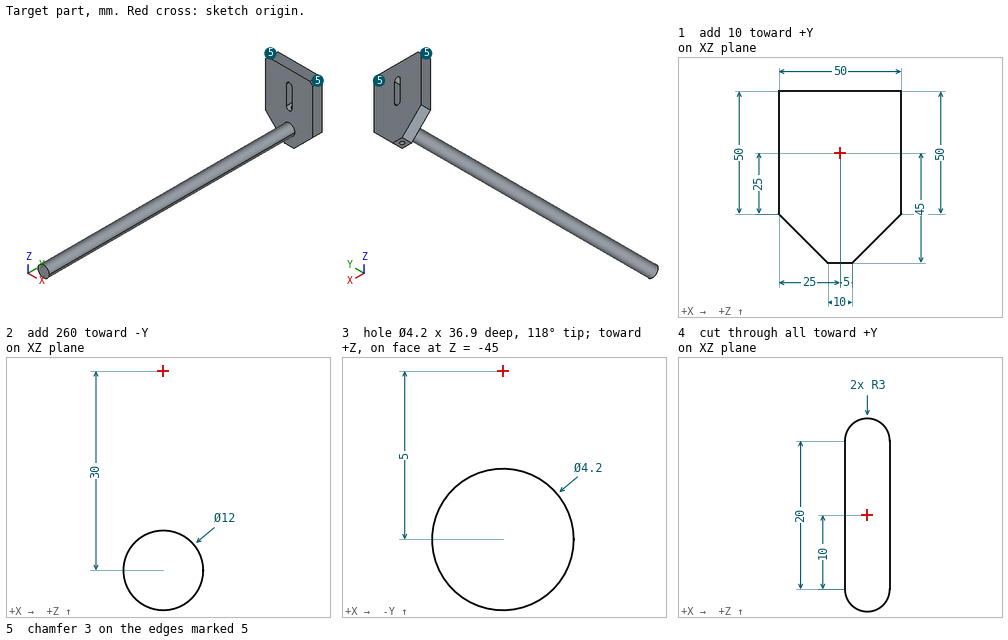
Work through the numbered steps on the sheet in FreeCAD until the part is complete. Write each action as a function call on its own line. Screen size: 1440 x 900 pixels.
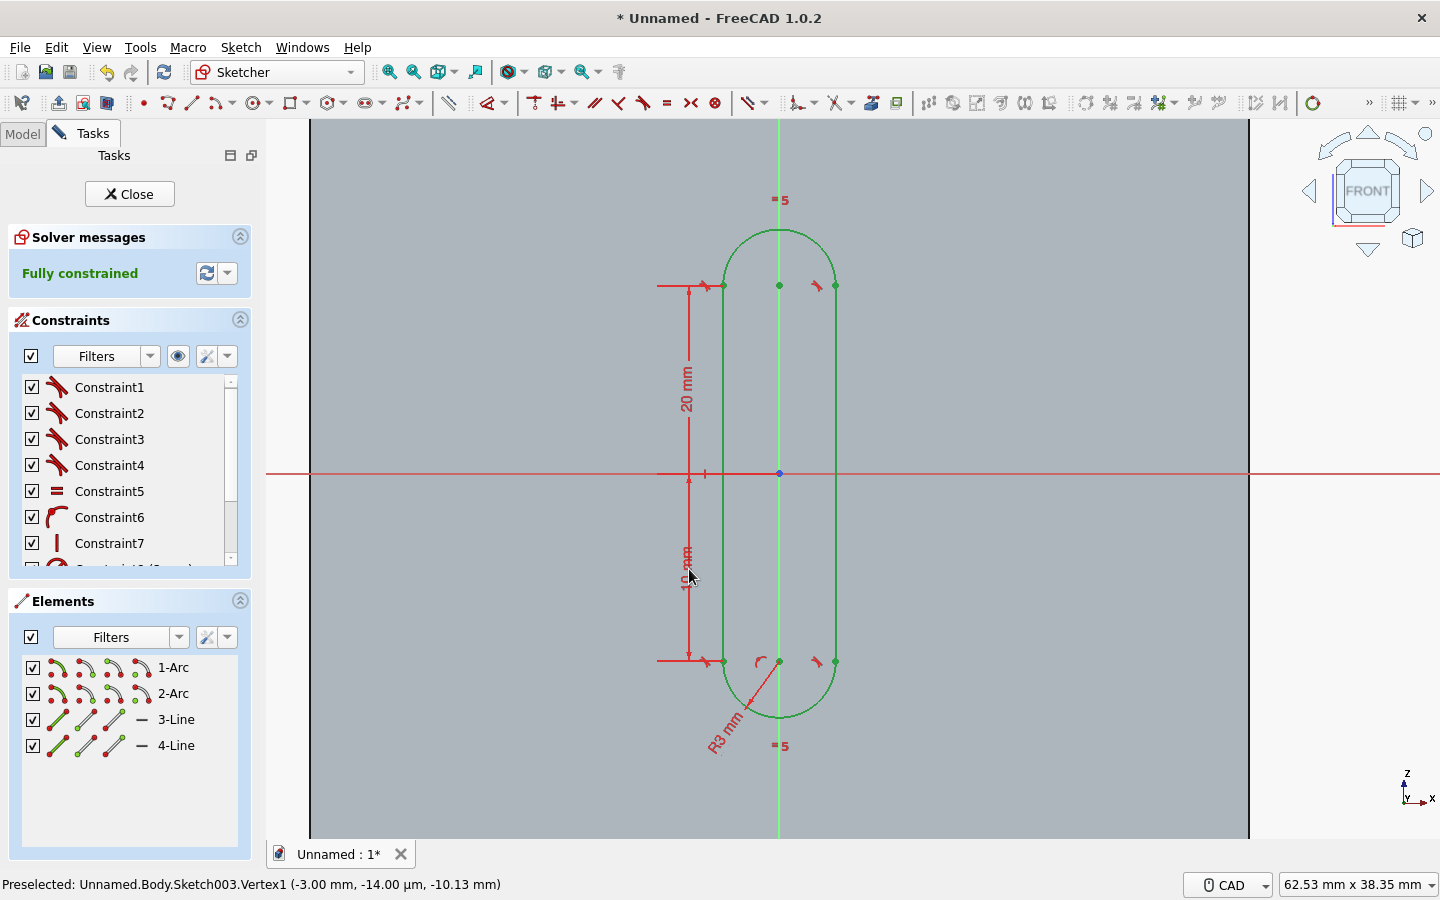
click(130, 194)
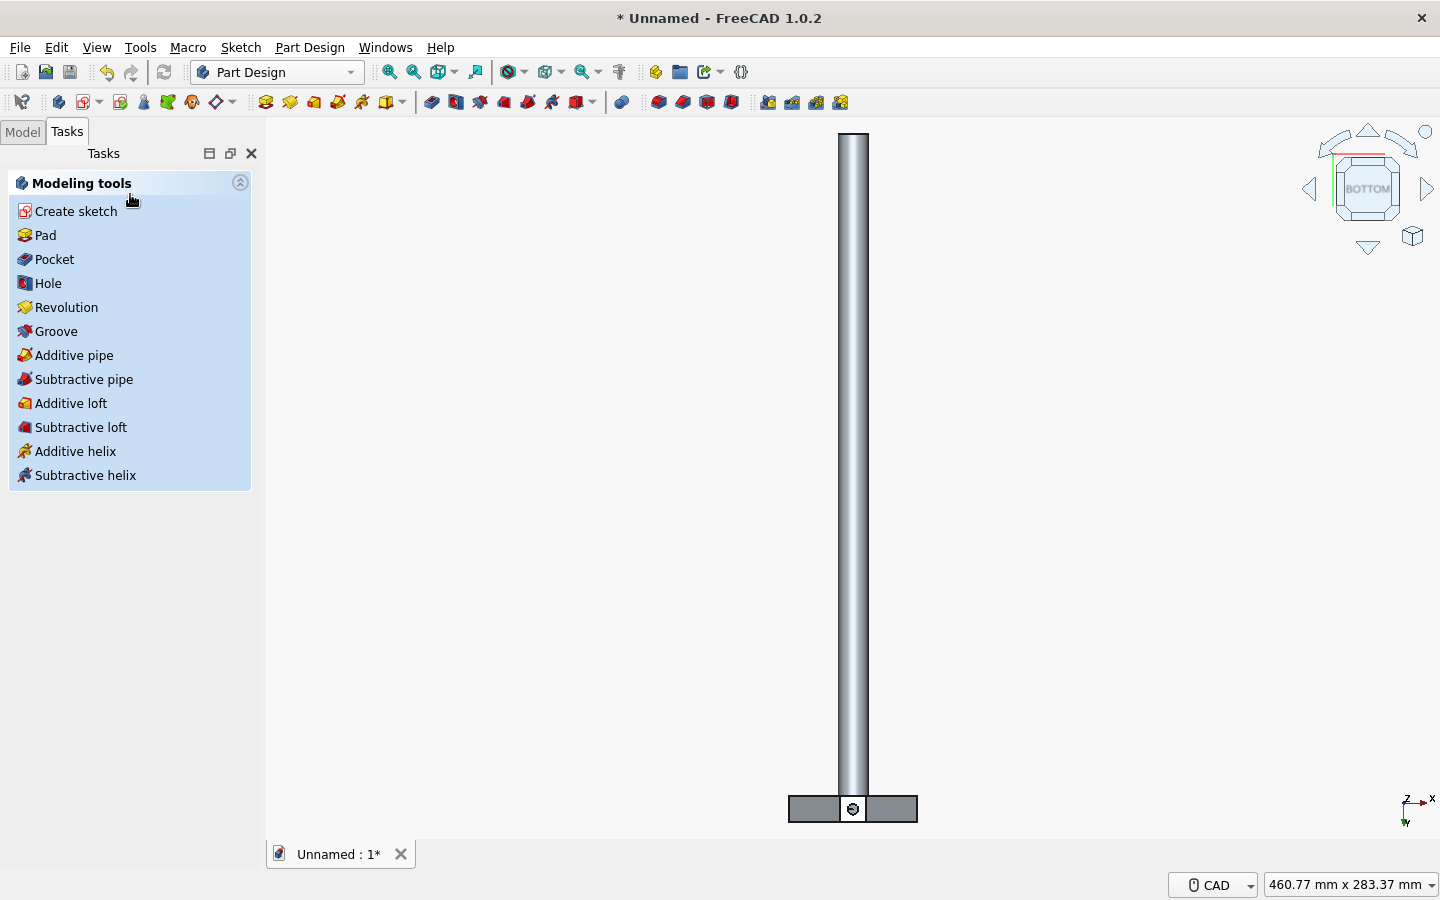
click(432, 102)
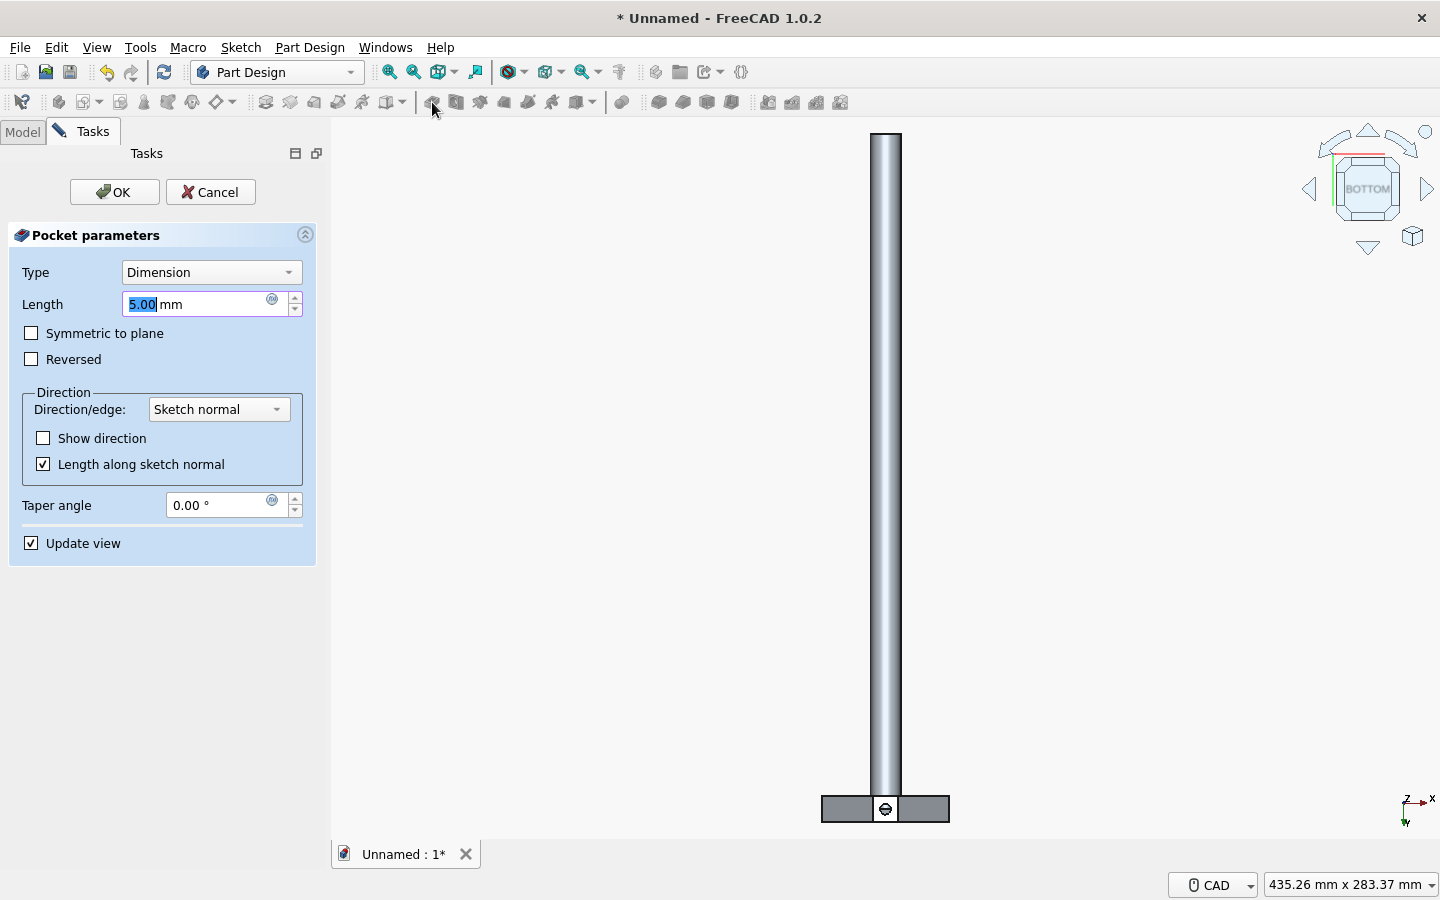
click(212, 272)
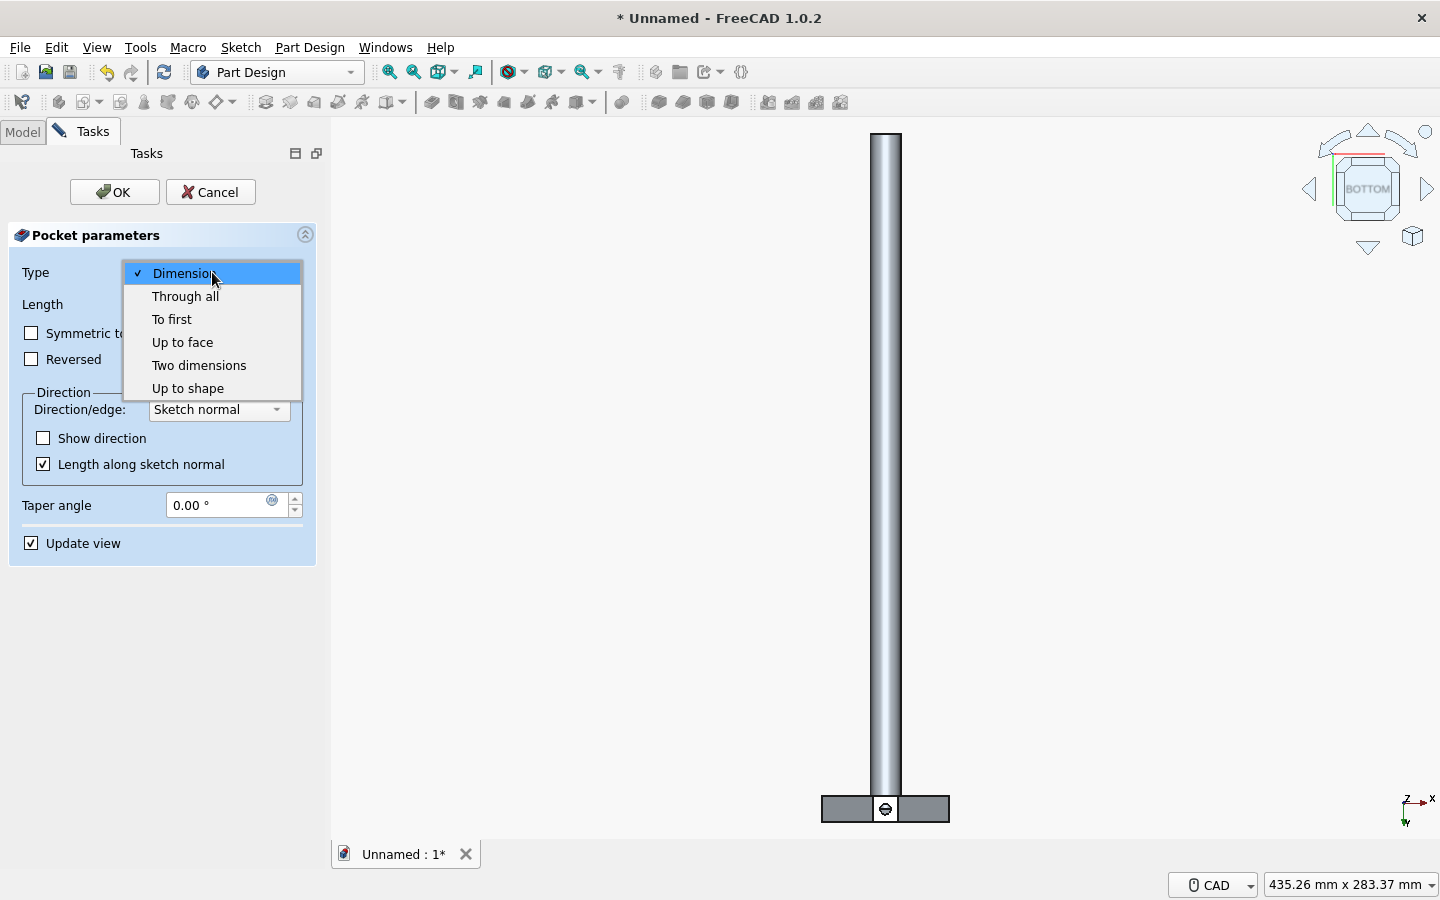
click(212, 296)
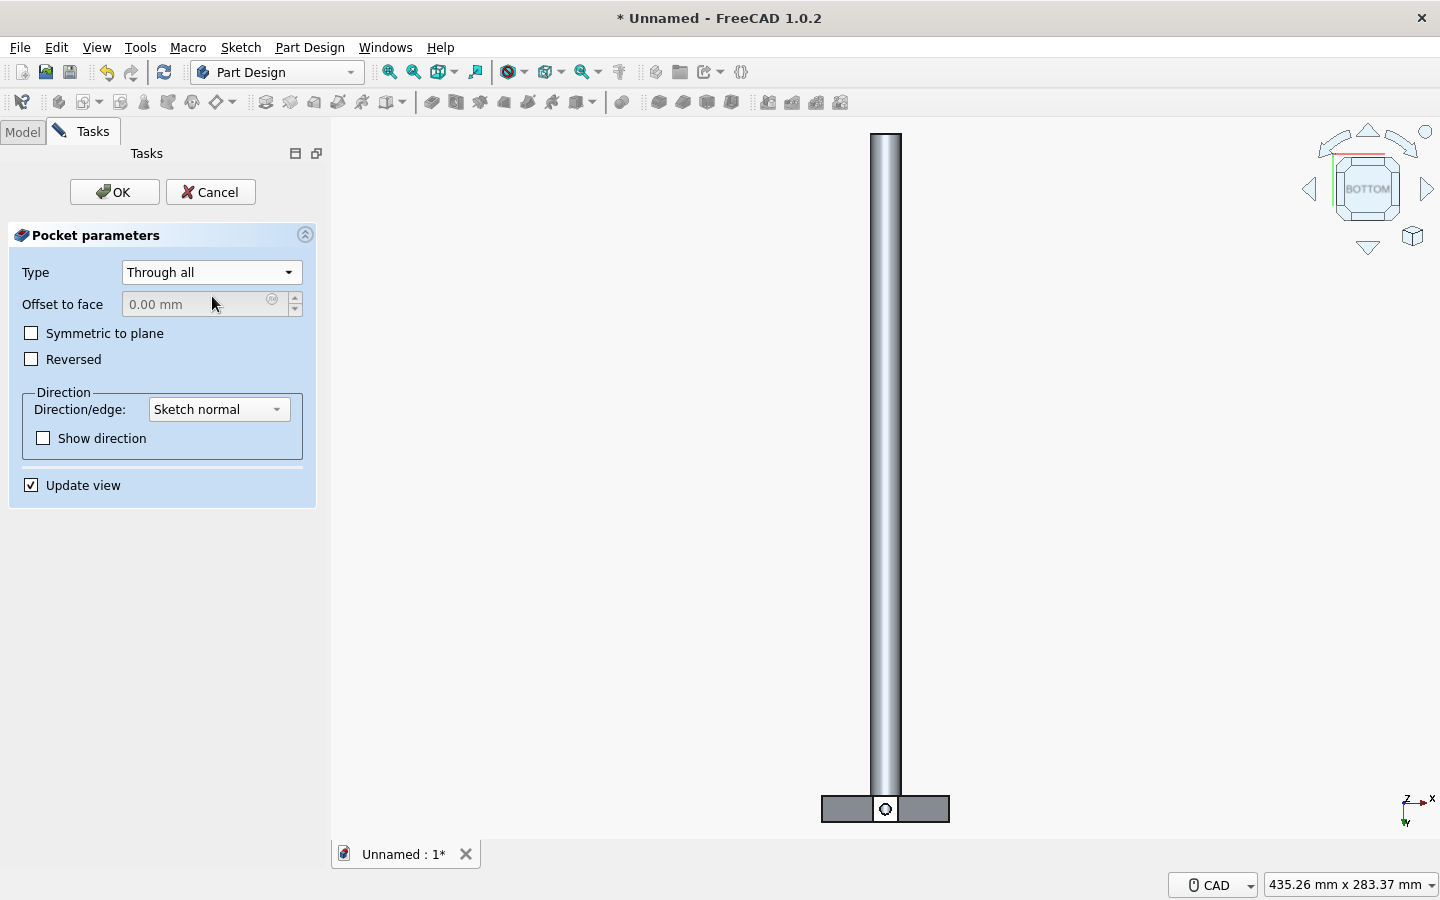
click(115, 192)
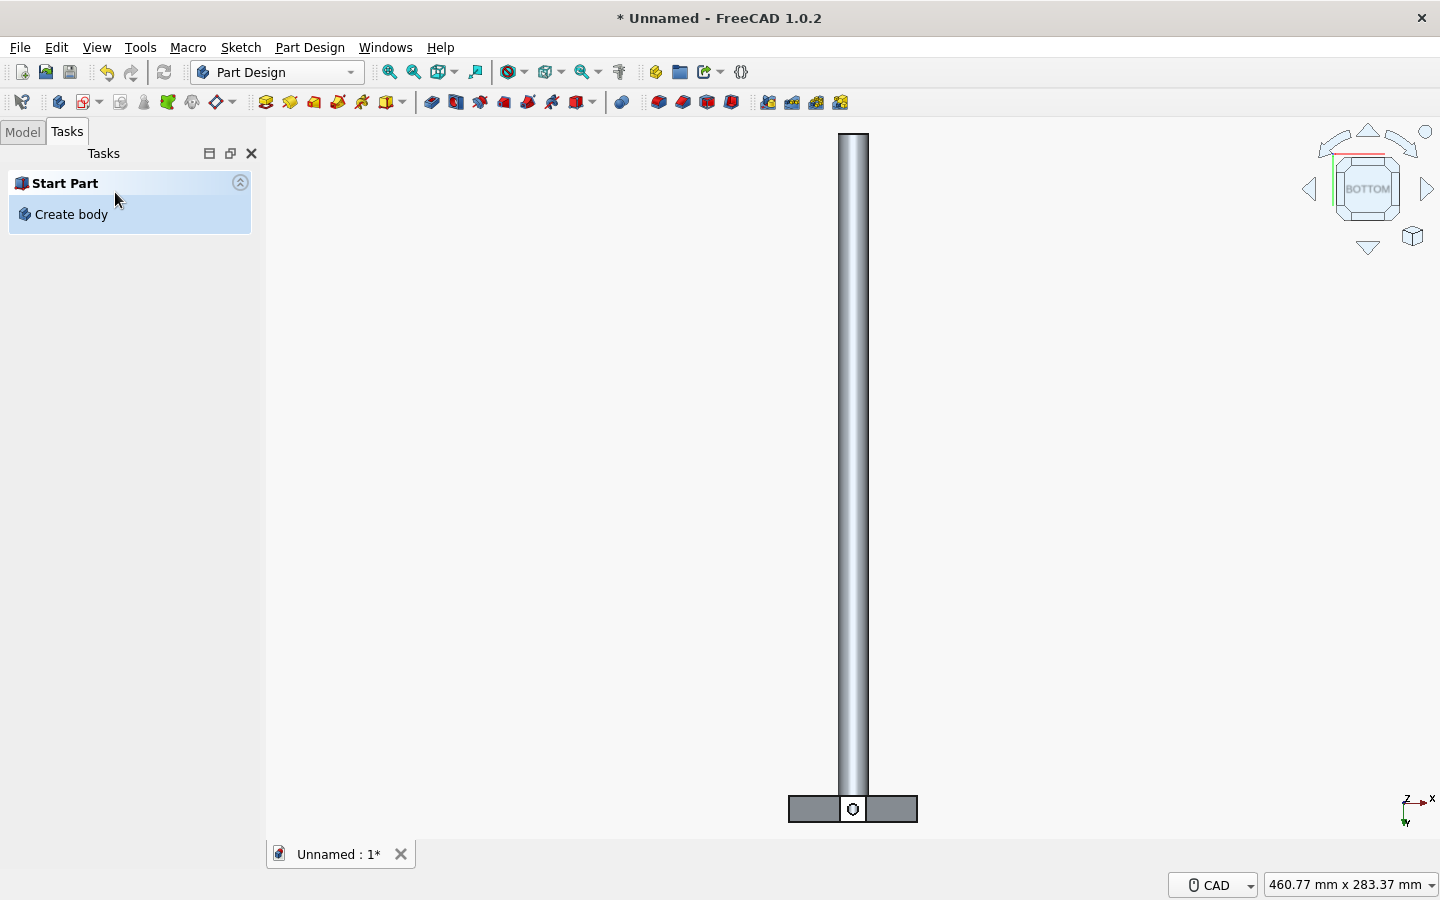
key(0)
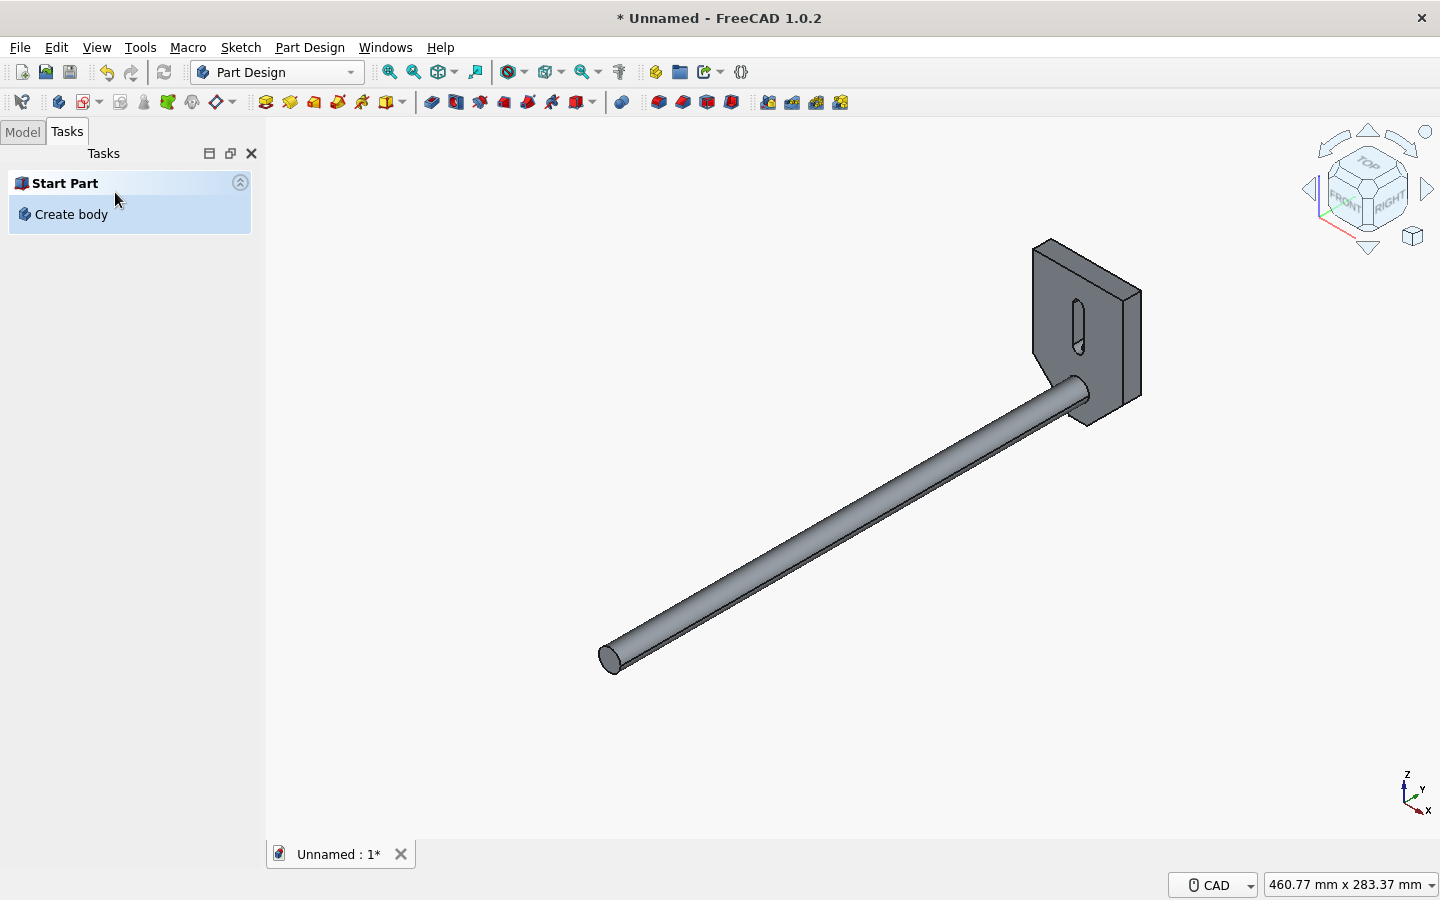
click(1132, 295)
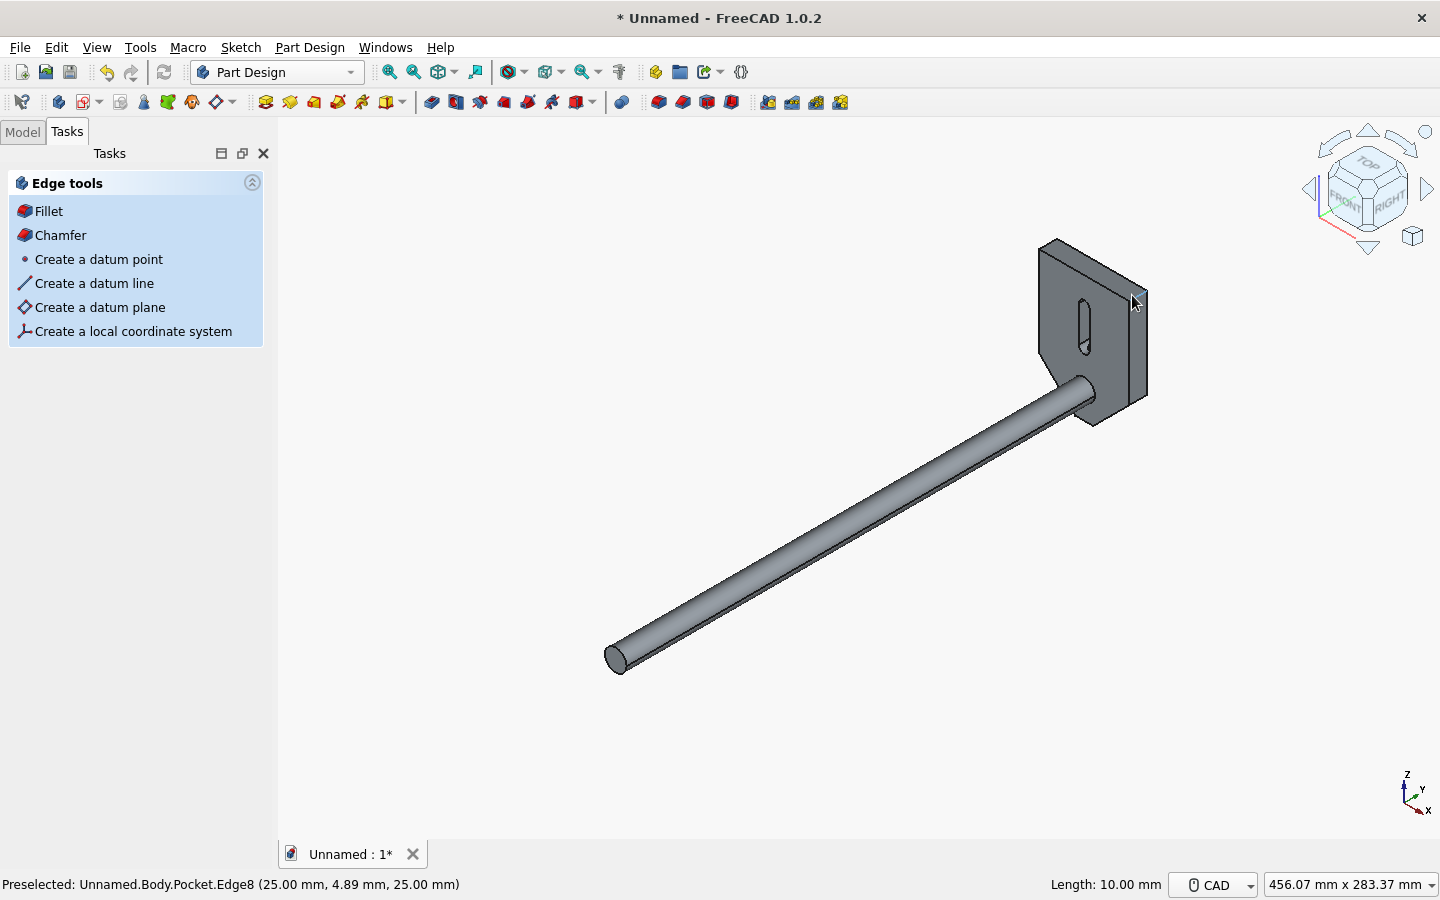
key(2)